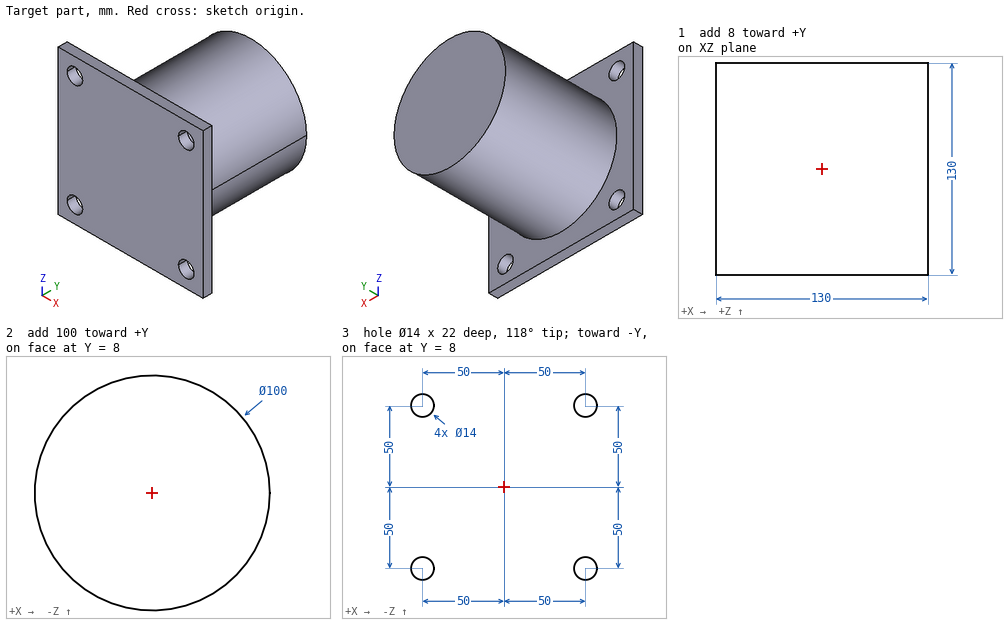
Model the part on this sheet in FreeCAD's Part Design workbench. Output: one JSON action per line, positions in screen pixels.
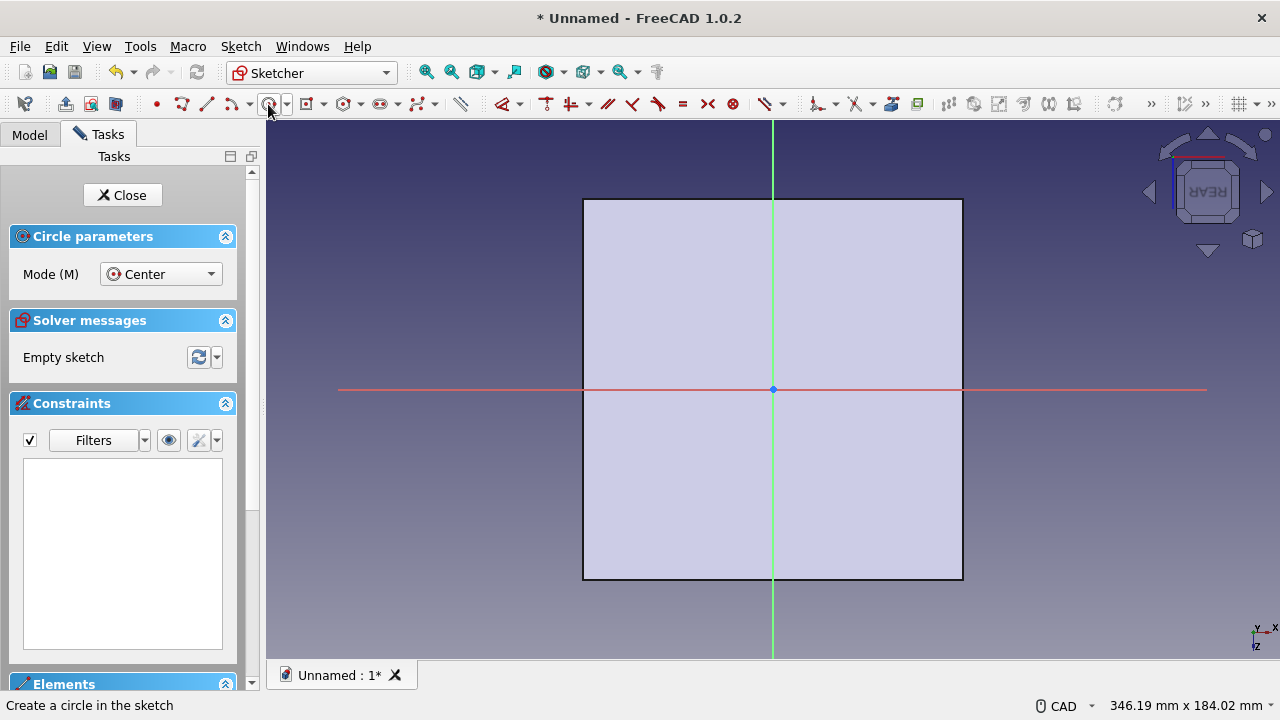
{"action": "left_click", "coordinate": [773, 389]}
{"action": "left_click", "coordinate": [877, 286]}
{"action": "key", "text": "Escape"}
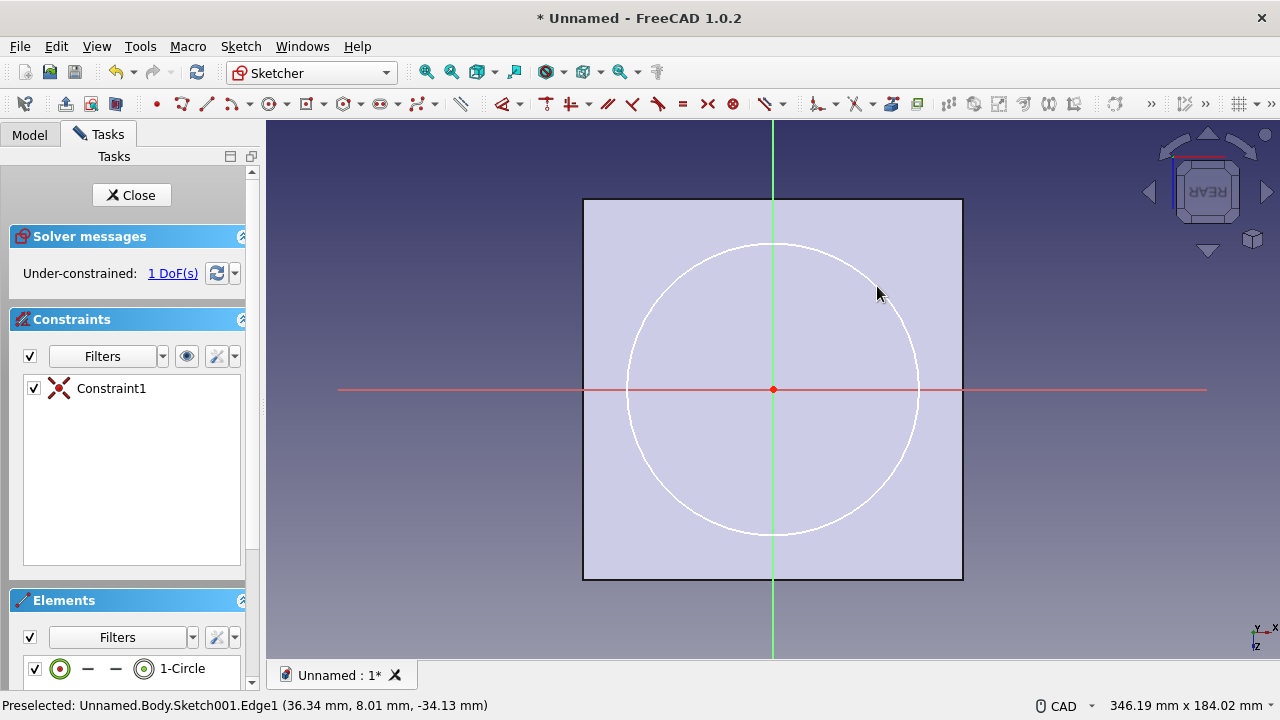
{"action": "left_click", "coordinate": [502, 104]}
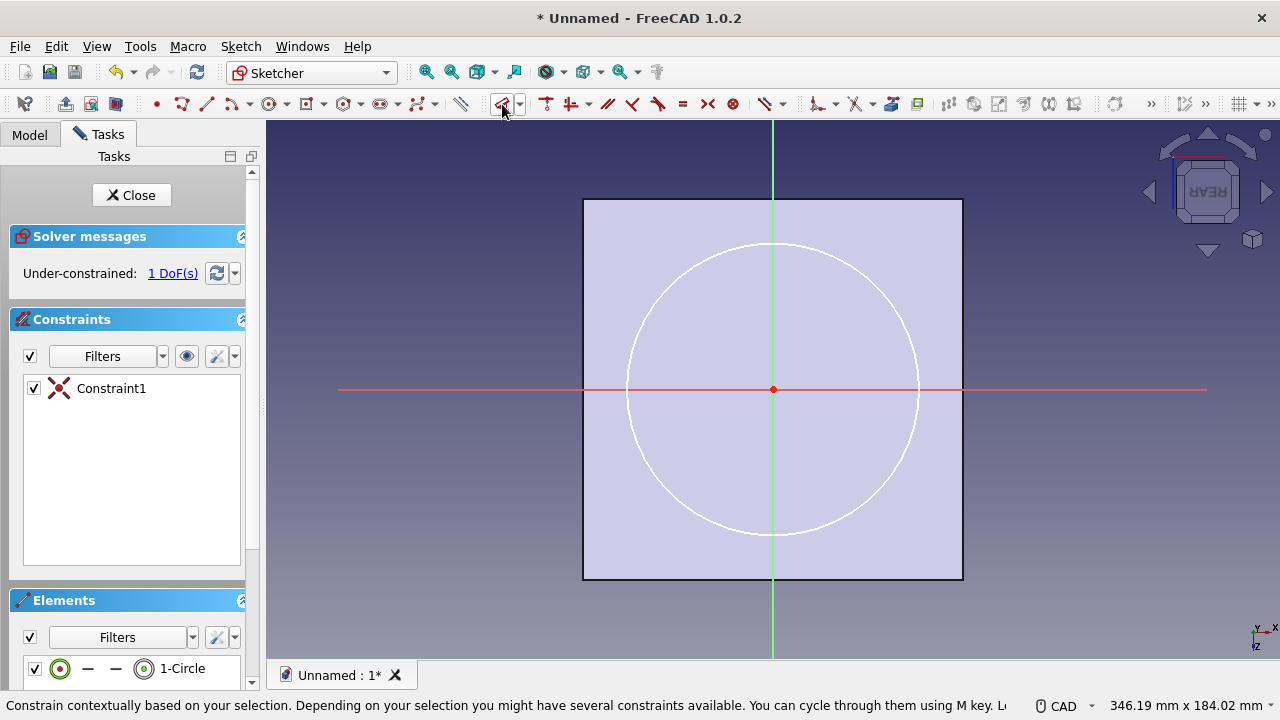
{"action": "left_click", "coordinate": [876, 286]}
{"action": "left_click", "coordinate": [899, 263]}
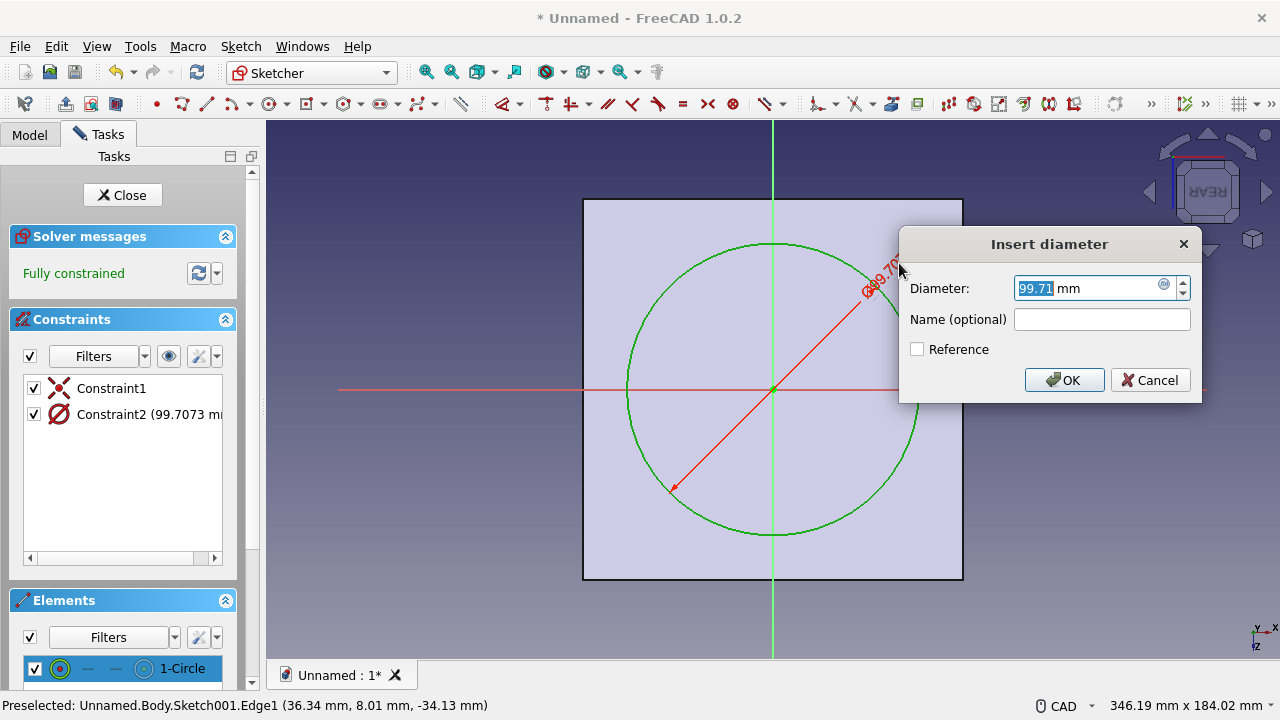
{"action": "type", "text": "100"}
{"action": "key", "text": "Return"}
{"action": "key", "text": "Escape"}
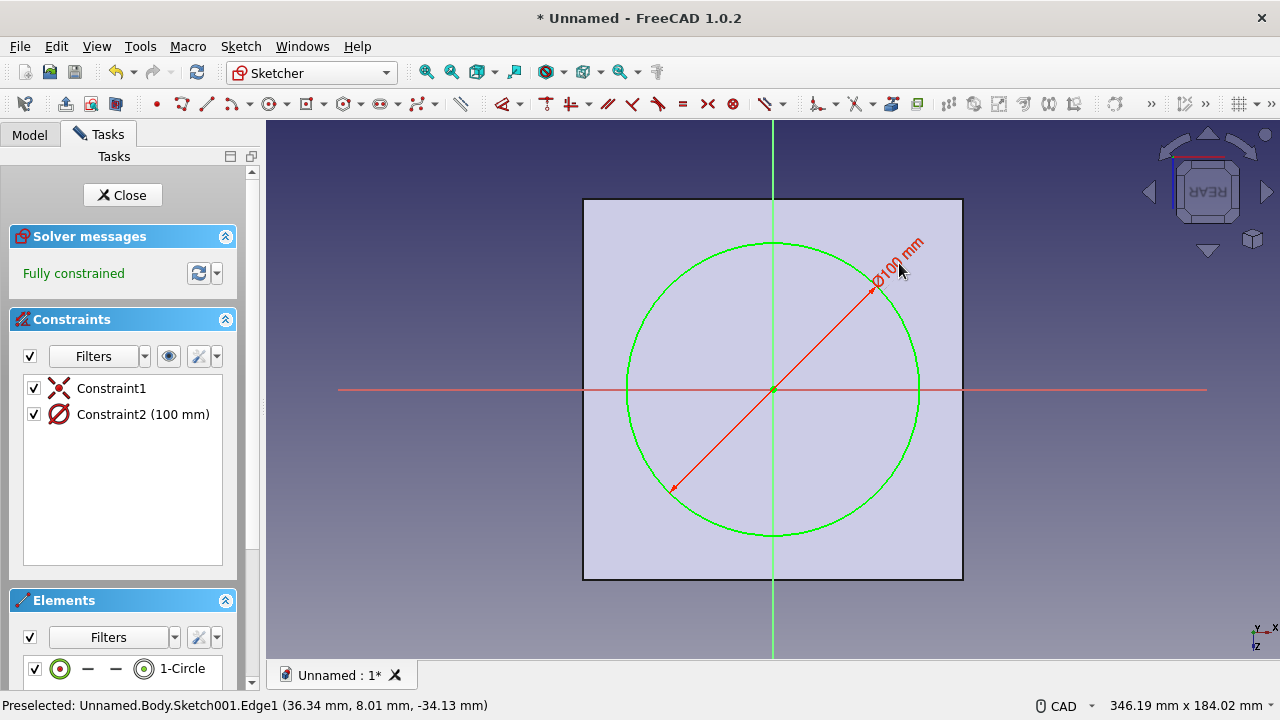
{"action": "left_click", "coordinate": [123, 195]}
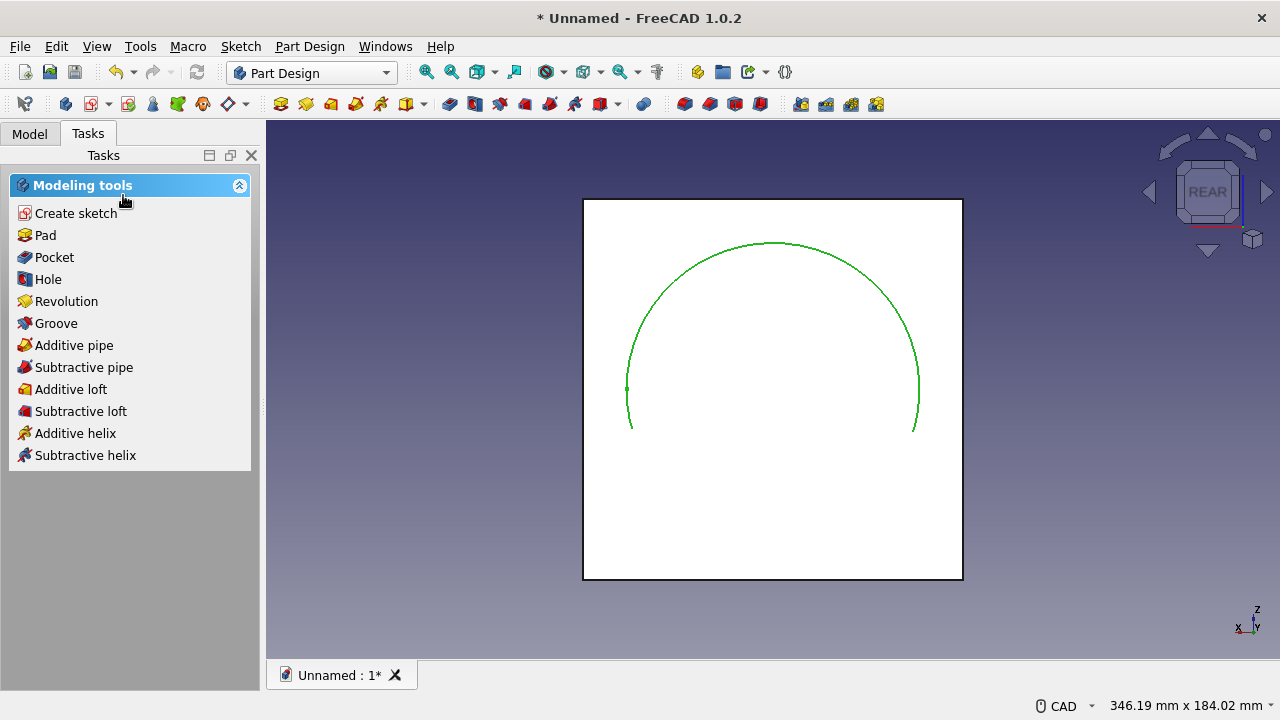
{"action": "left_click", "coordinate": [281, 104]}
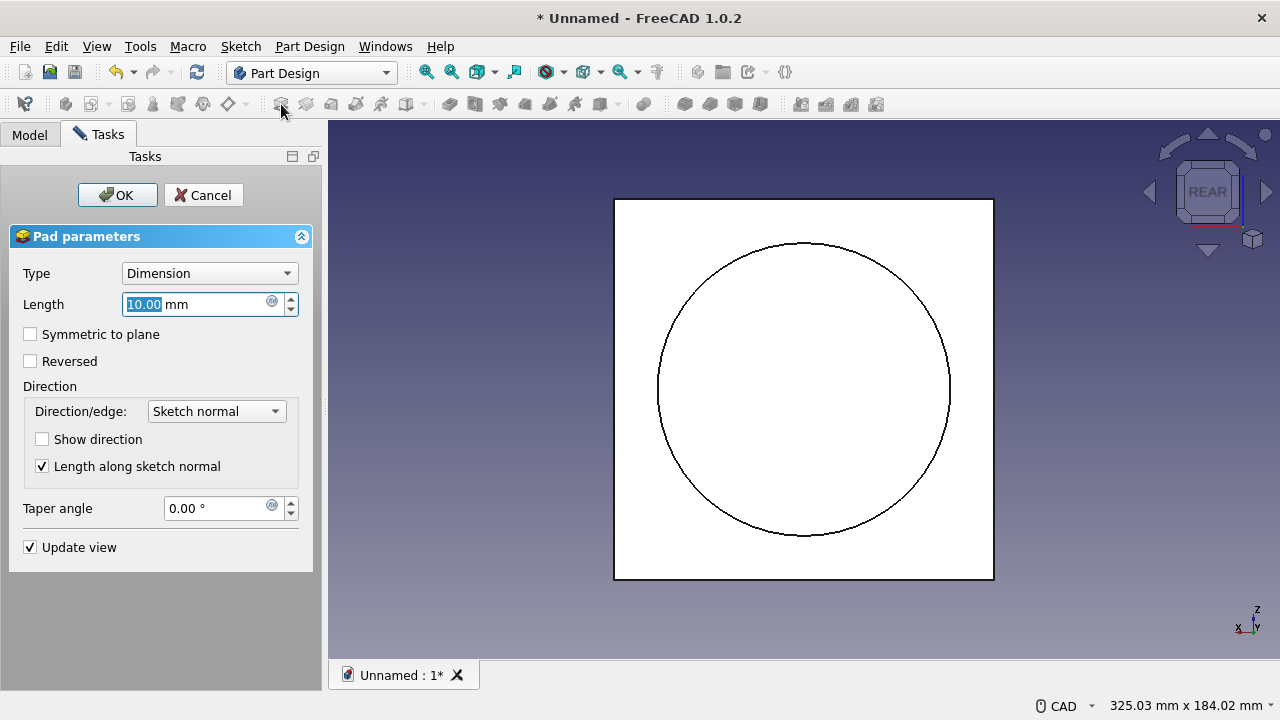
{"action": "type", "text": "100"}
{"action": "key", "text": "Tab"}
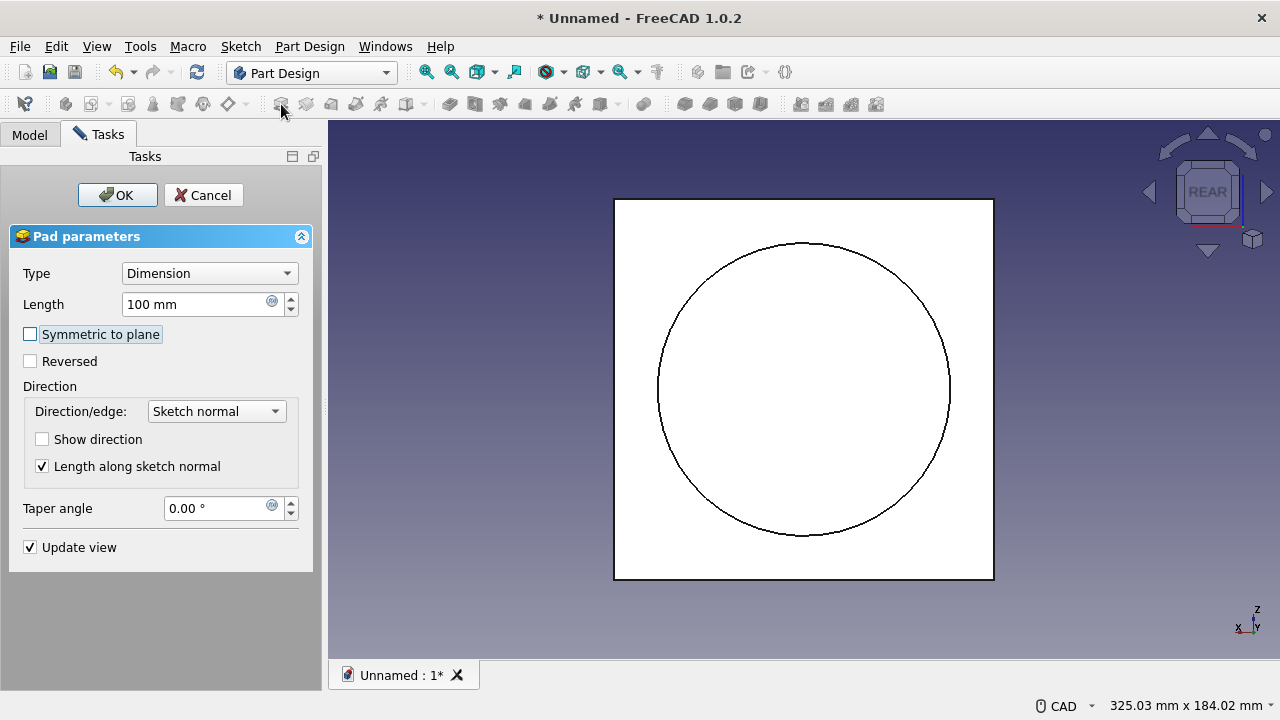
{"action": "left_click", "coordinate": [118, 195]}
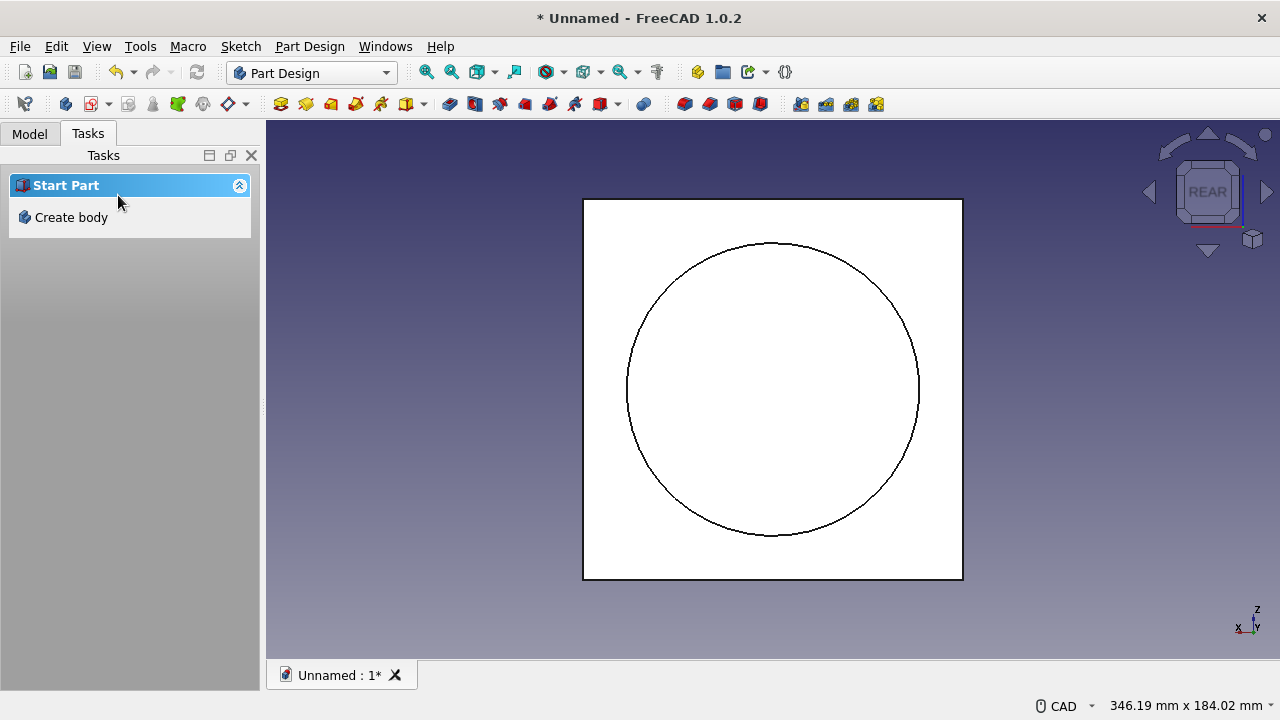
{"action": "left_click", "coordinate": [610, 225]}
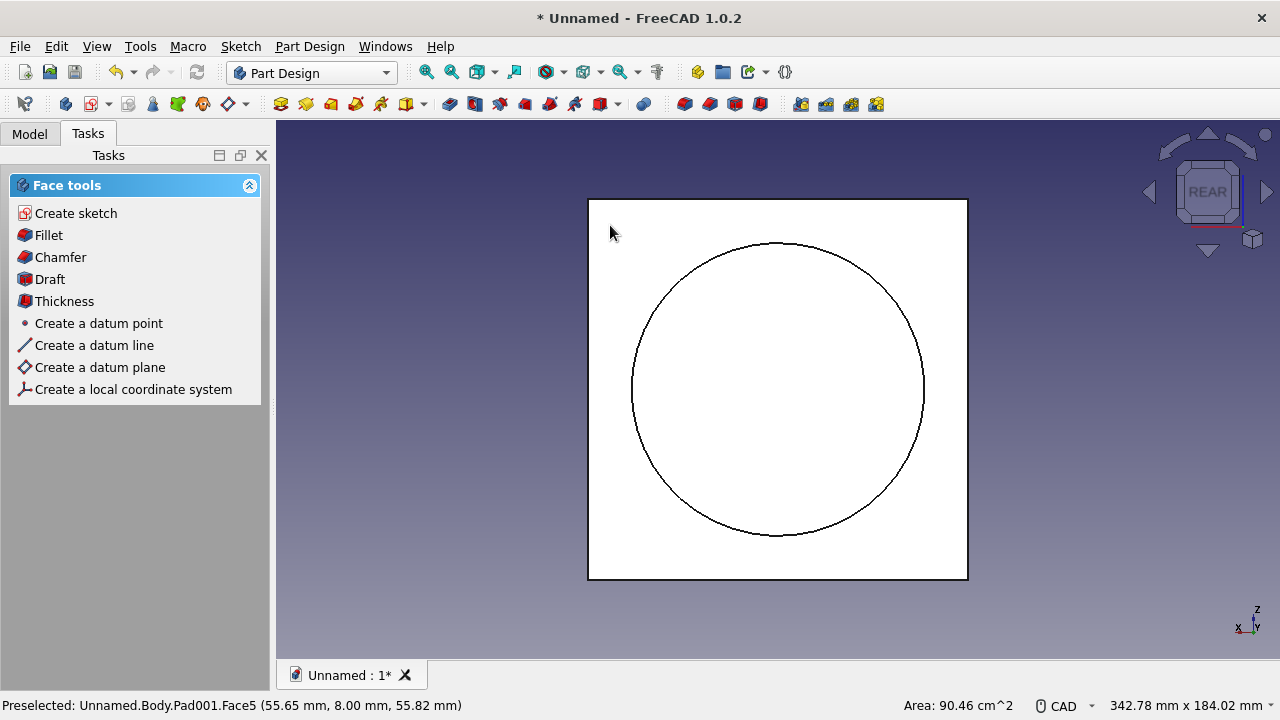
{"action": "left_click", "coordinate": [90, 104]}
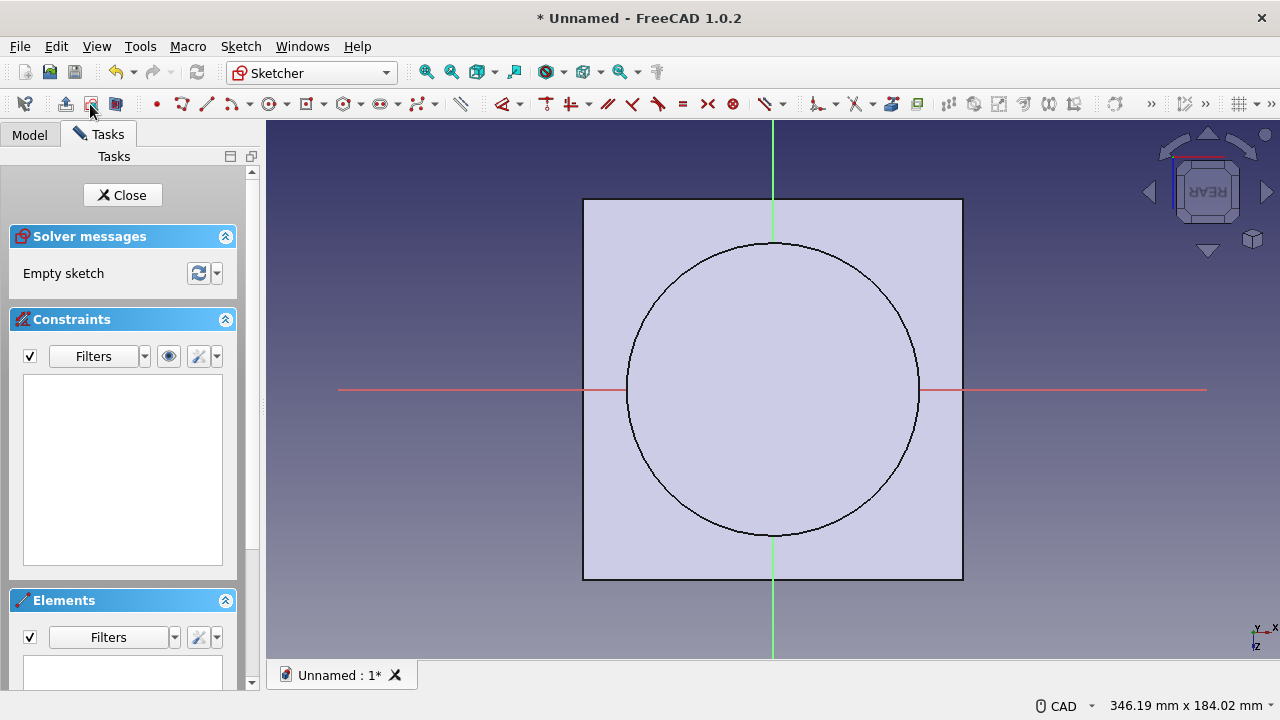
{"action": "left_click", "coordinate": [268, 104]}